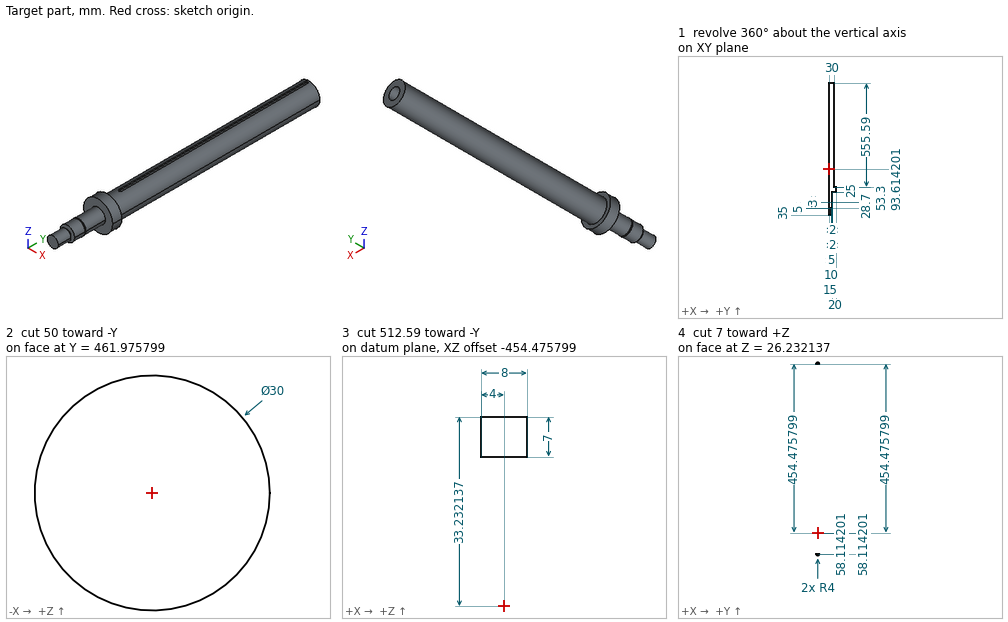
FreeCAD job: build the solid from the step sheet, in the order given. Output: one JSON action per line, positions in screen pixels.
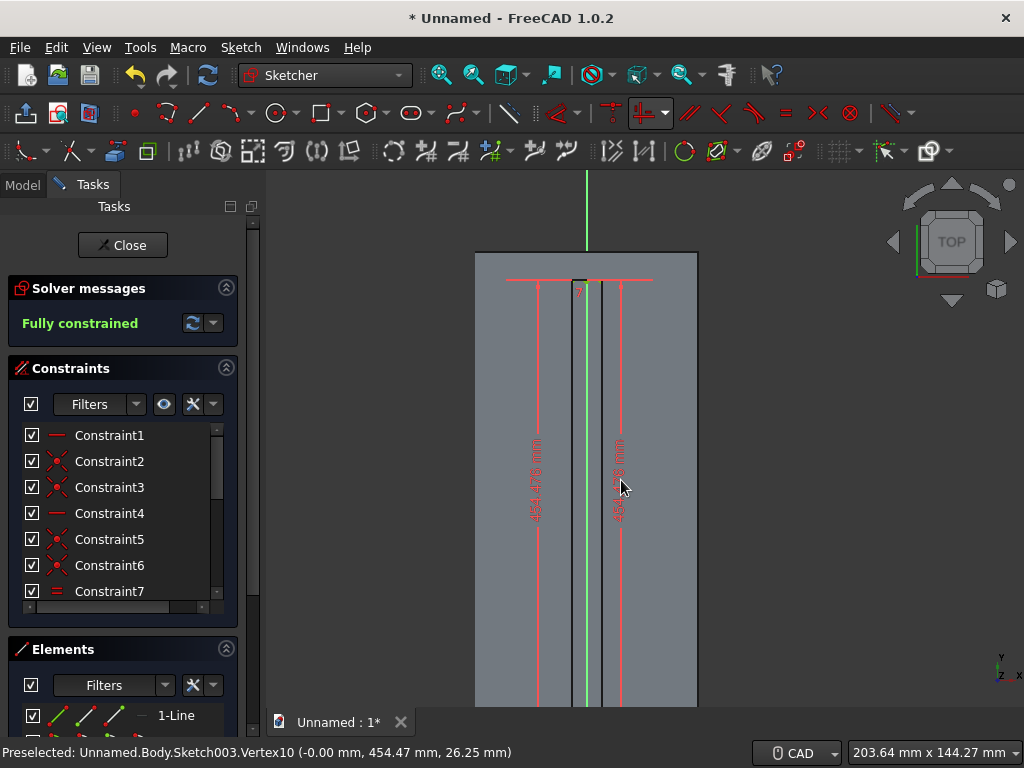
{"action": "left_click", "coordinate": [123, 245]}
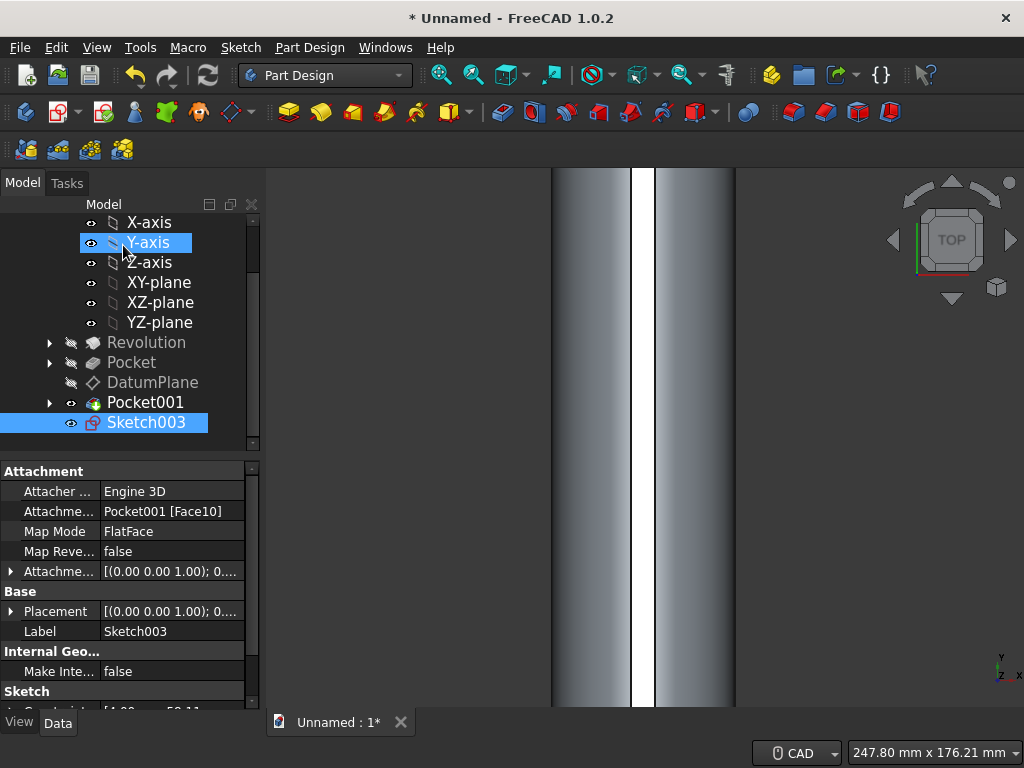
{"action": "left_click", "coordinate": [504, 112]}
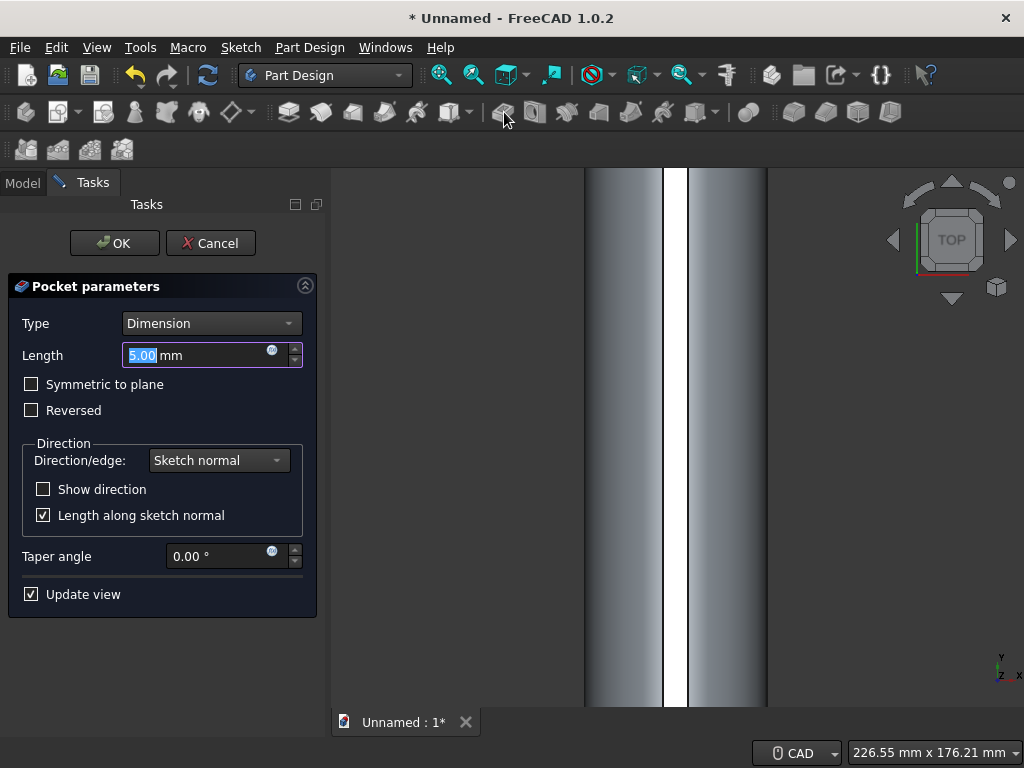
{"action": "type", "text": "7"}
{"action": "key", "text": "Tab"}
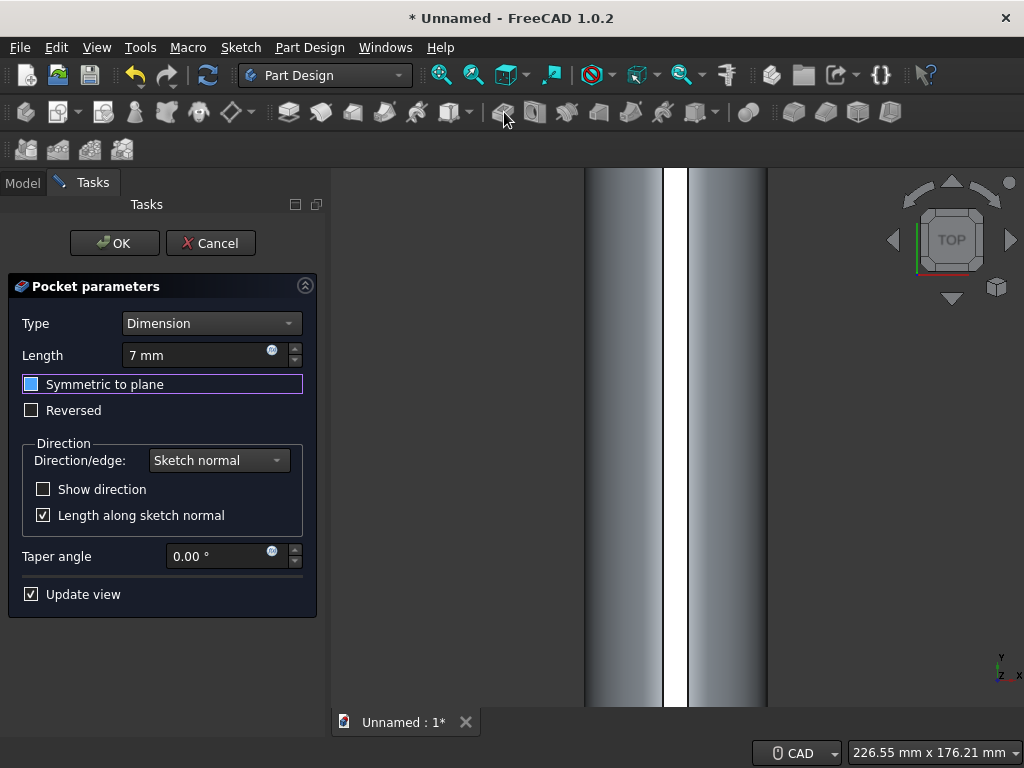
{"action": "left_click", "coordinate": [30, 410]}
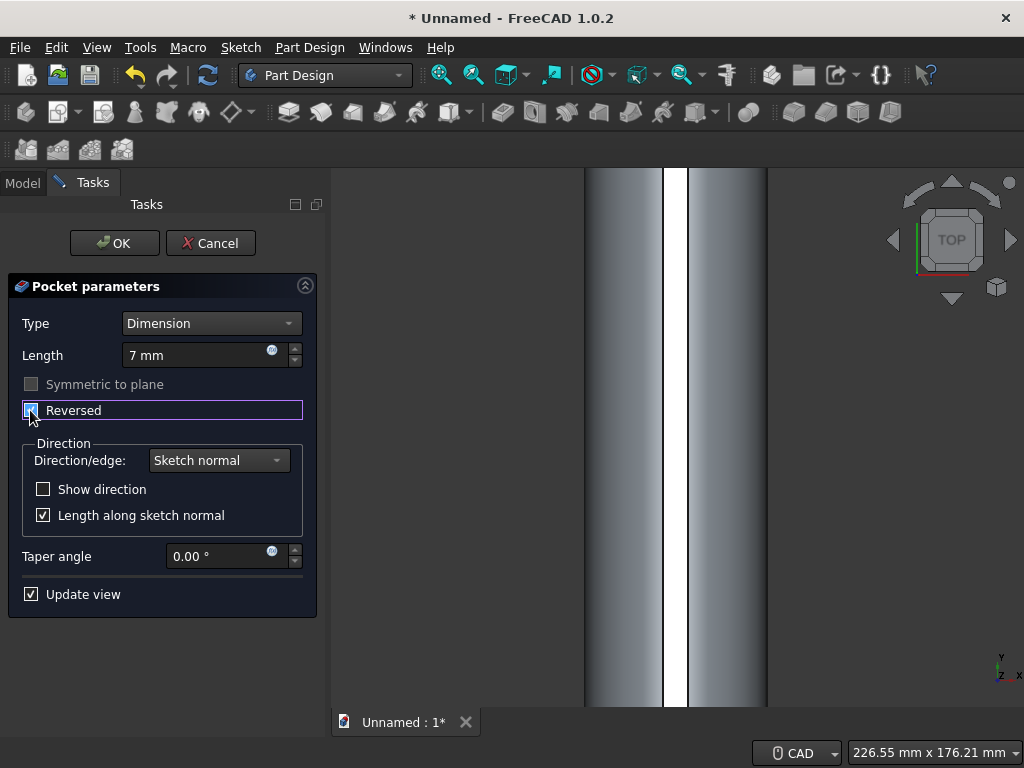
{"action": "left_click", "coordinate": [115, 243]}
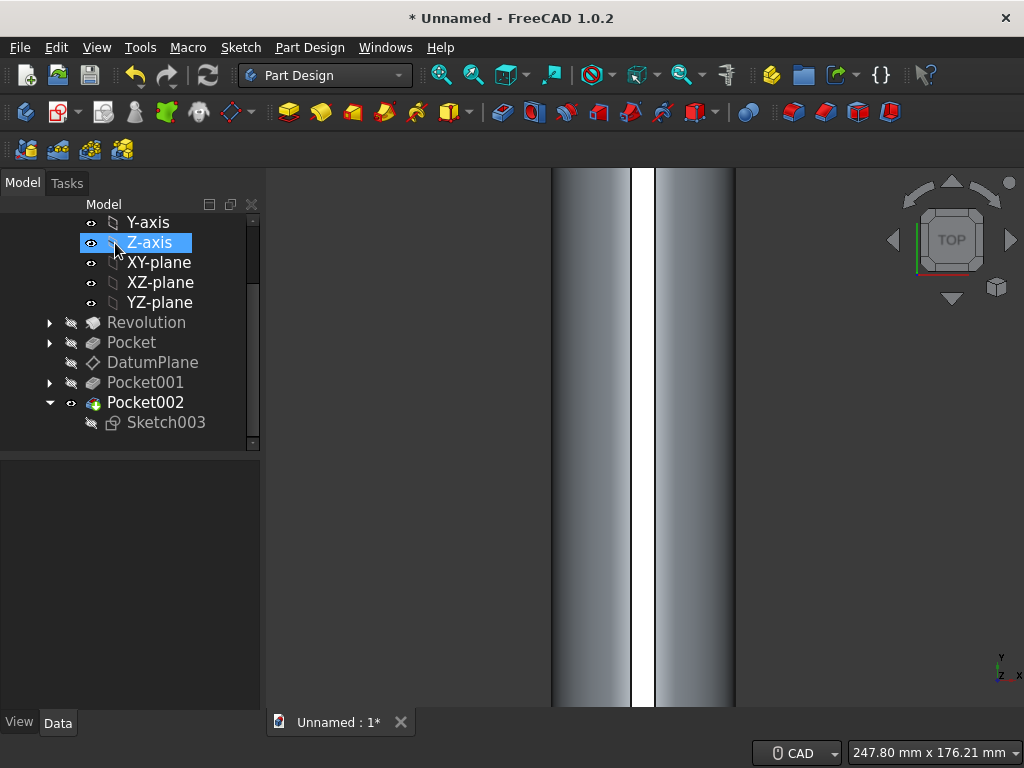
{"action": "key", "text": "0"}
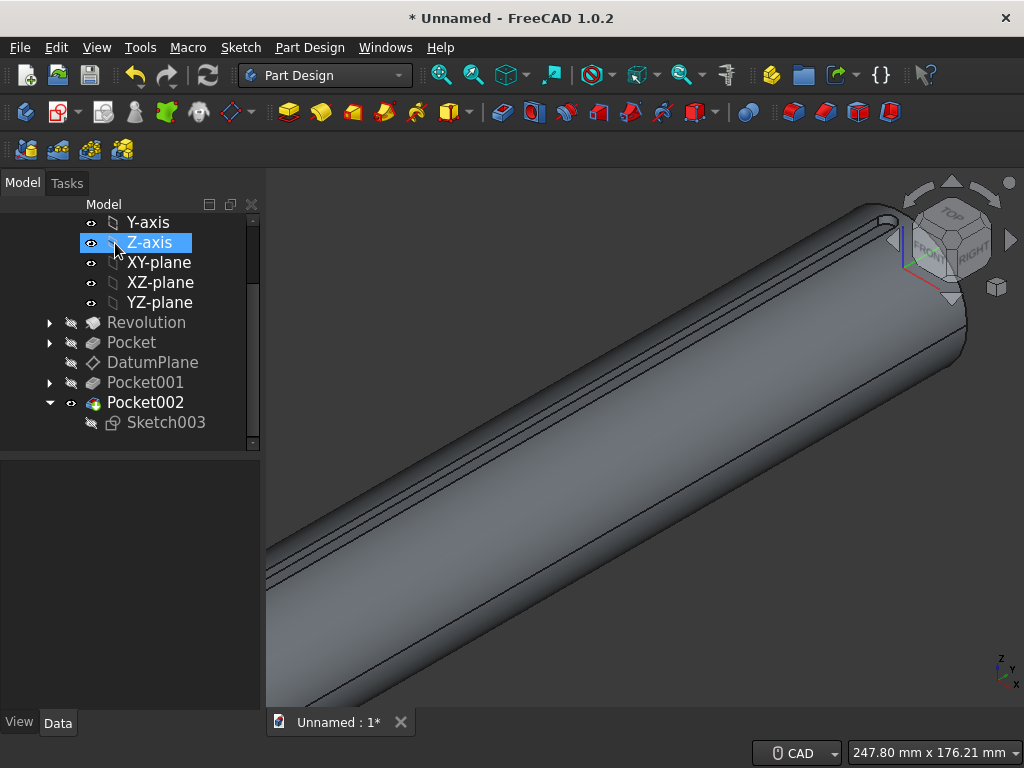
{"action": "key", "text": "v f"}